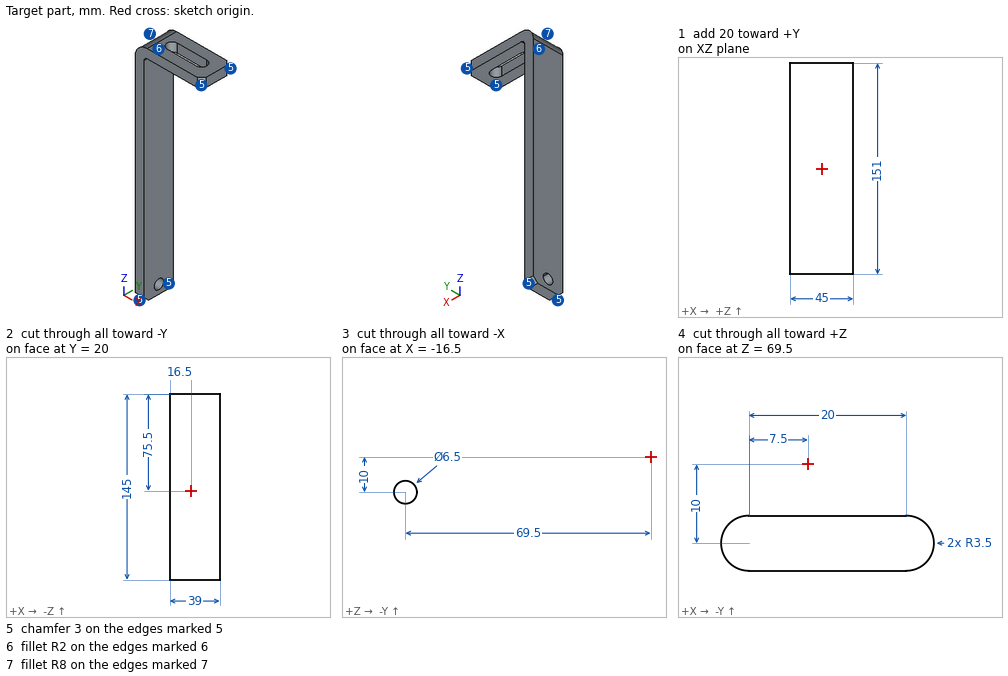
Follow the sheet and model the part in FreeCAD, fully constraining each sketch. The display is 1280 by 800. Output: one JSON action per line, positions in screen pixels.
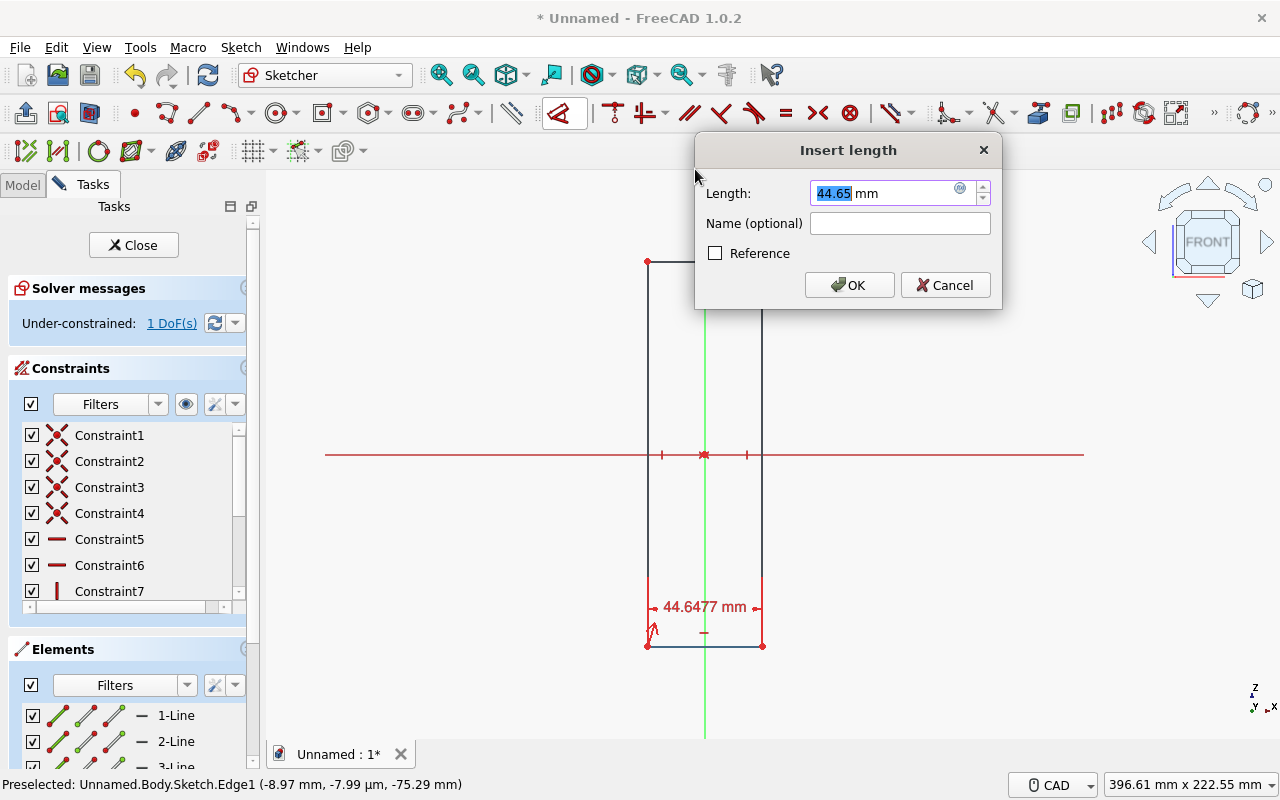
{"action": "type", "text": "45"}
{"action": "key", "text": "Return"}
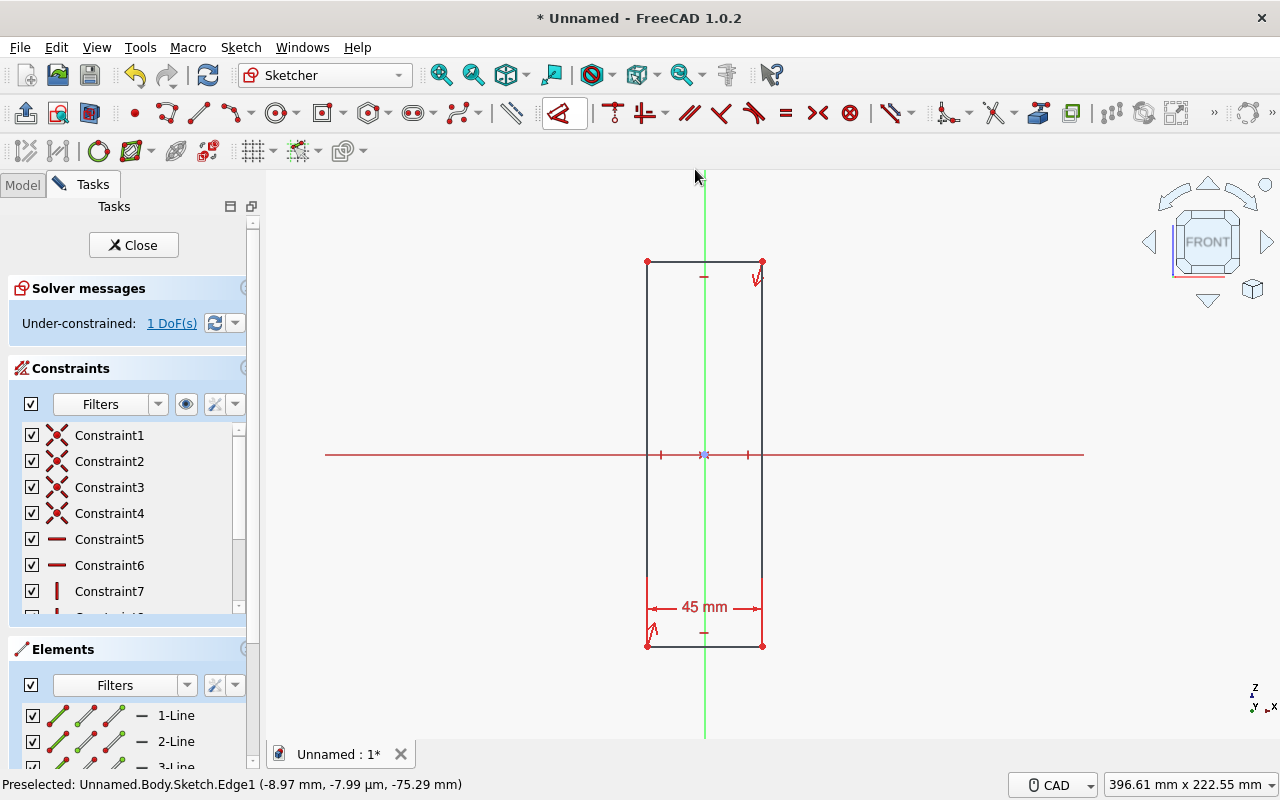
{"action": "left_click", "coordinate": [762, 531]}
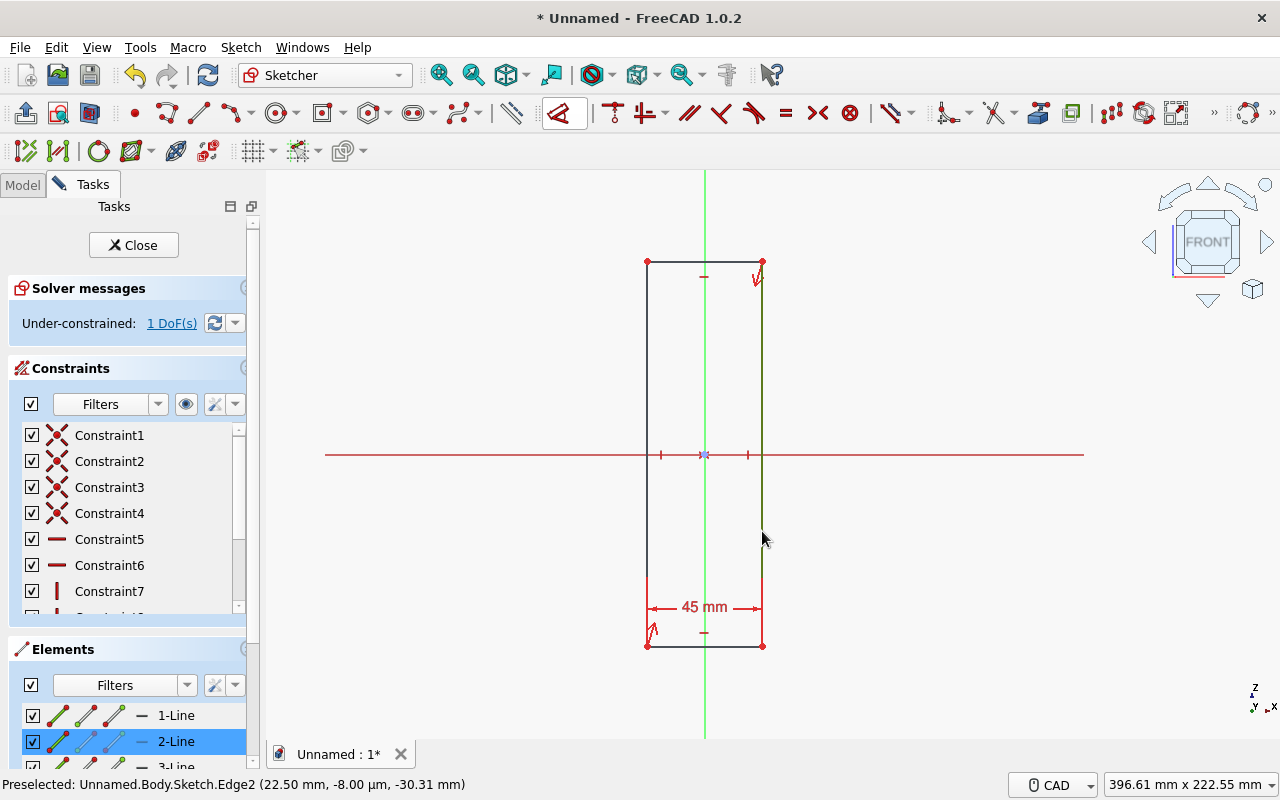
{"action": "left_click", "coordinate": [582, 114]}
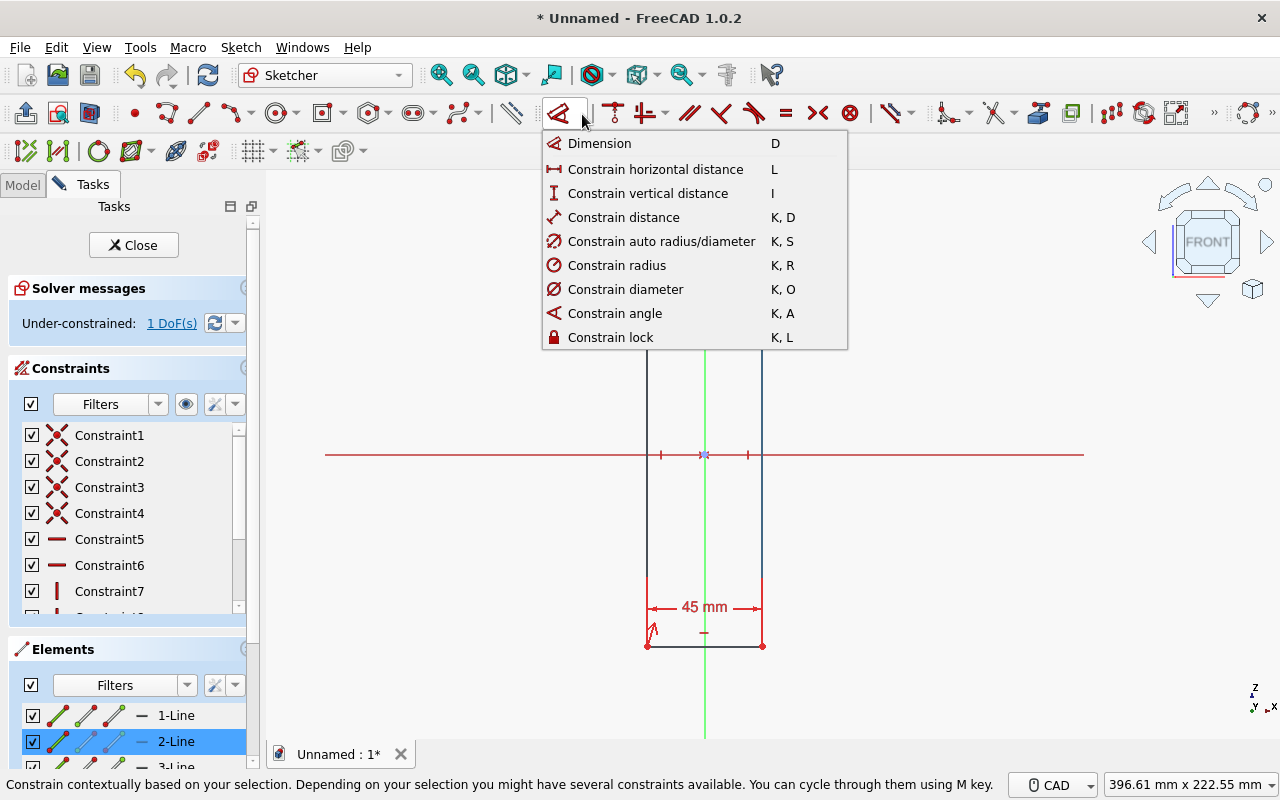
{"action": "left_click", "coordinate": [695, 193]}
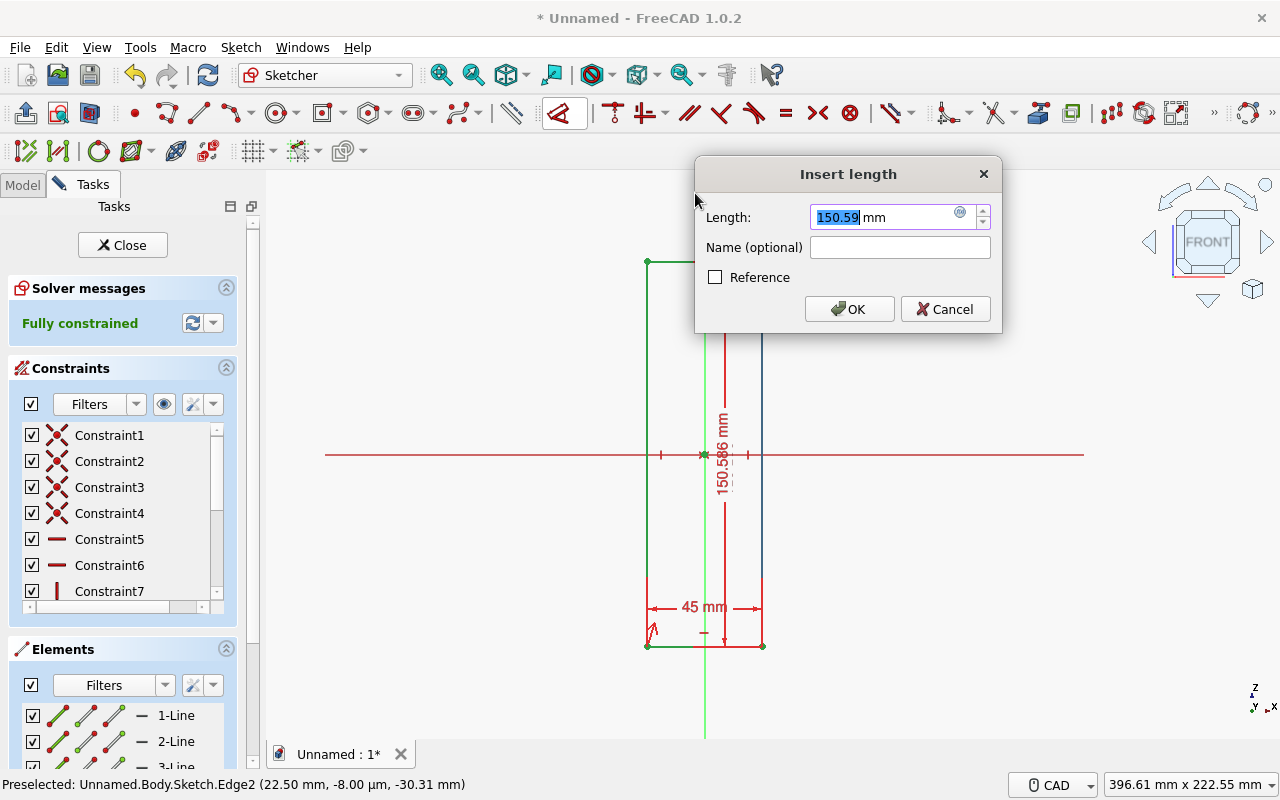
{"action": "type", "text": "151"}
{"action": "key", "text": "Return"}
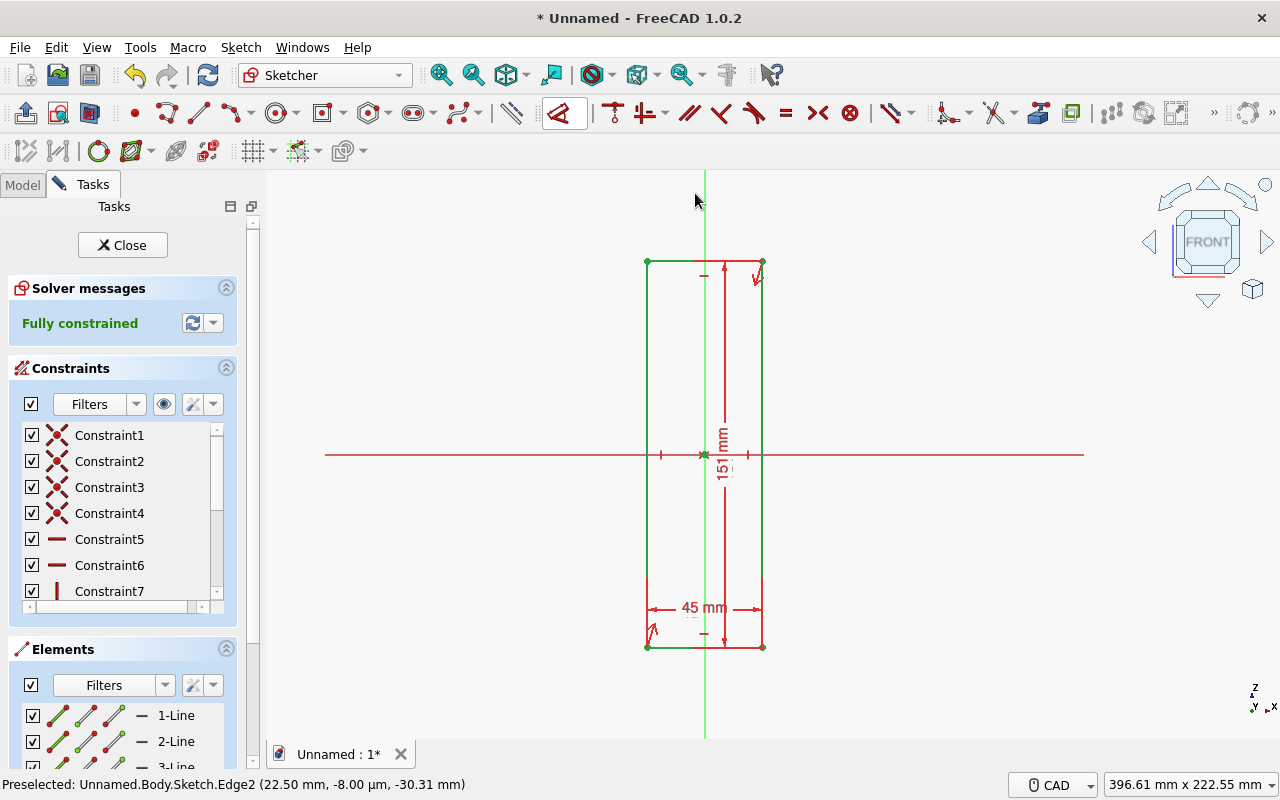
{"action": "left_click", "coordinate": [123, 245]}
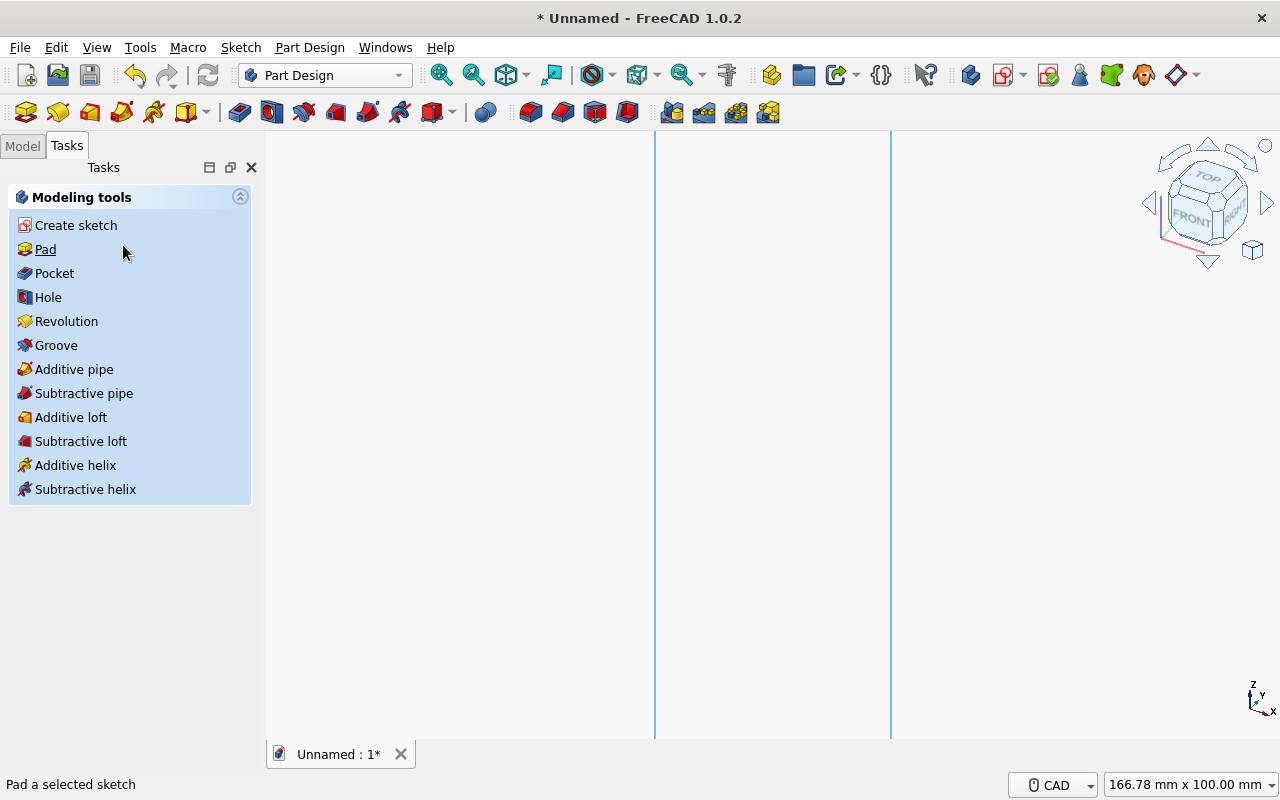
{"action": "left_click", "coordinate": [26, 112]}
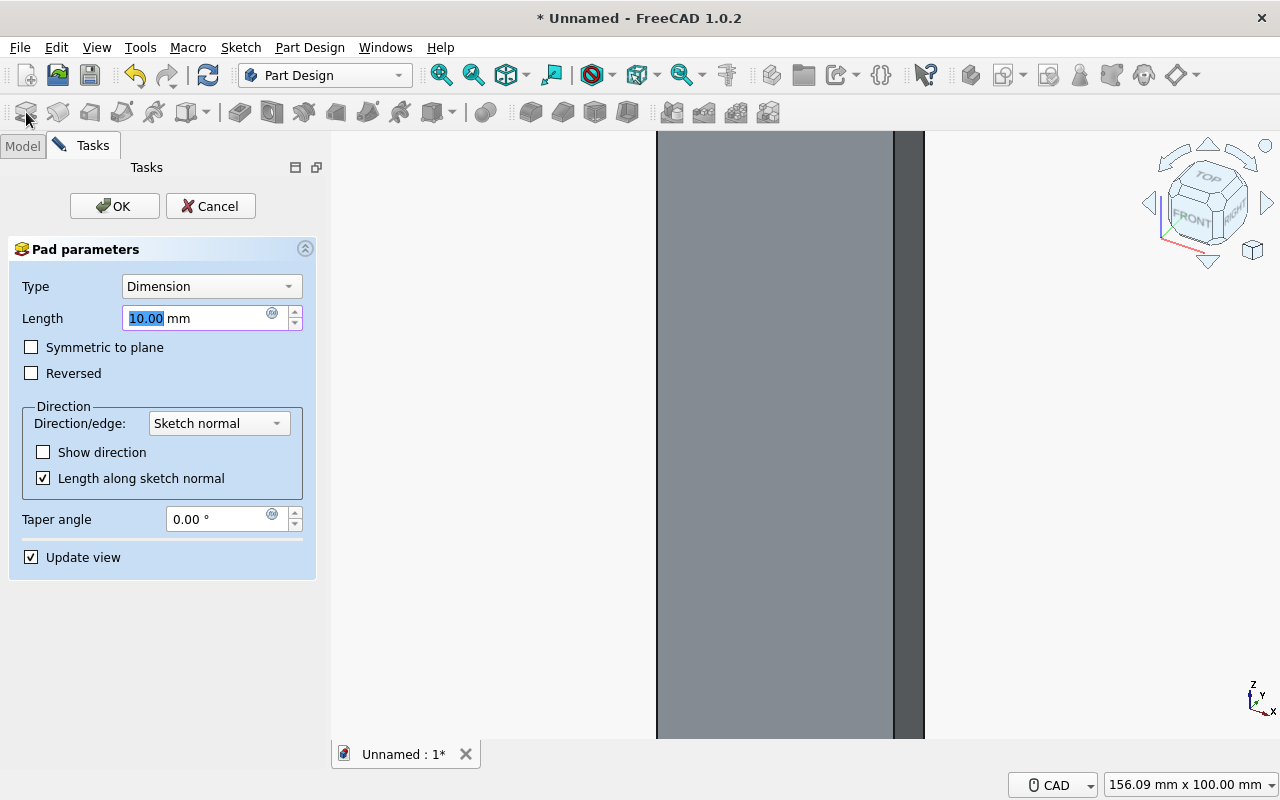
{"action": "type", "text": "20"}
{"action": "key", "text": "Tab"}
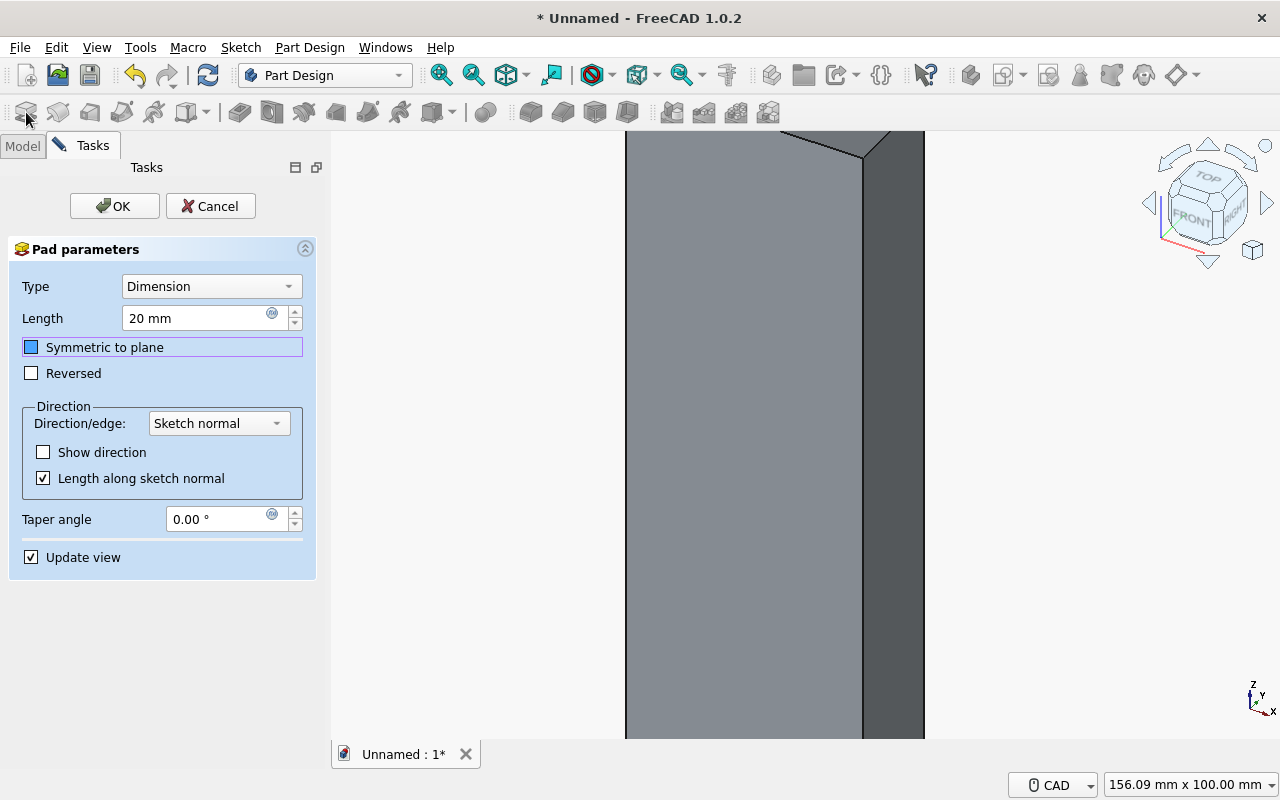
{"action": "left_click", "coordinate": [30, 373]}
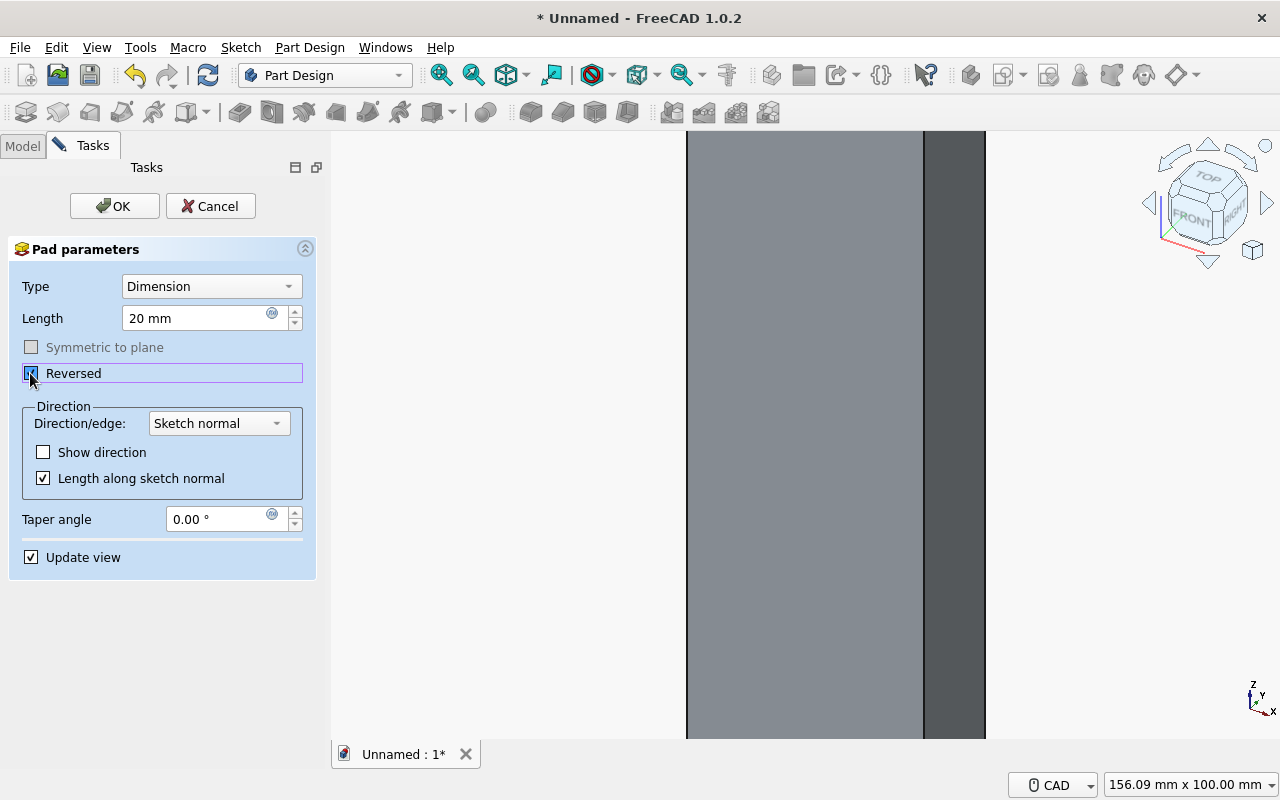
{"action": "left_click", "coordinate": [115, 206]}